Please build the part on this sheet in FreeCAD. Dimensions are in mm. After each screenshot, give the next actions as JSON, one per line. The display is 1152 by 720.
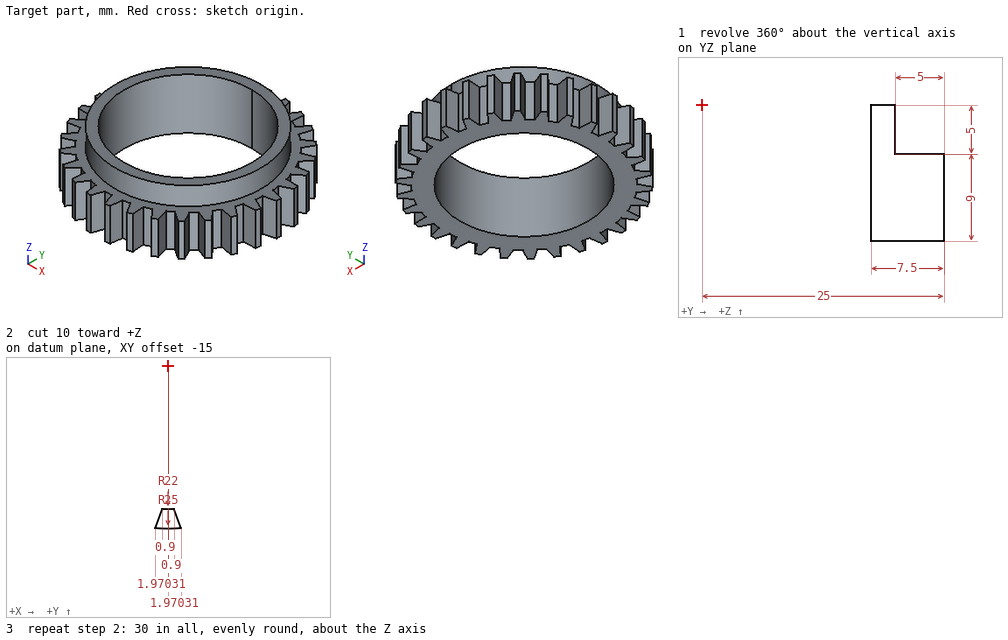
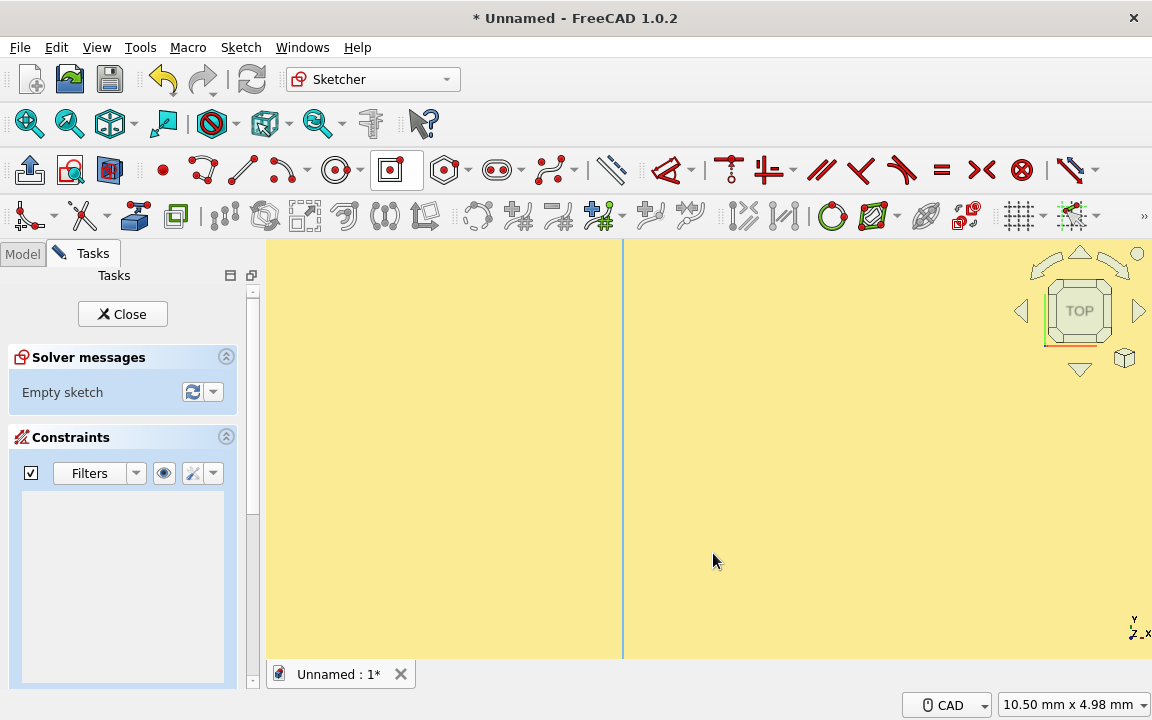
{"action": "left_click", "coordinate": [244, 170]}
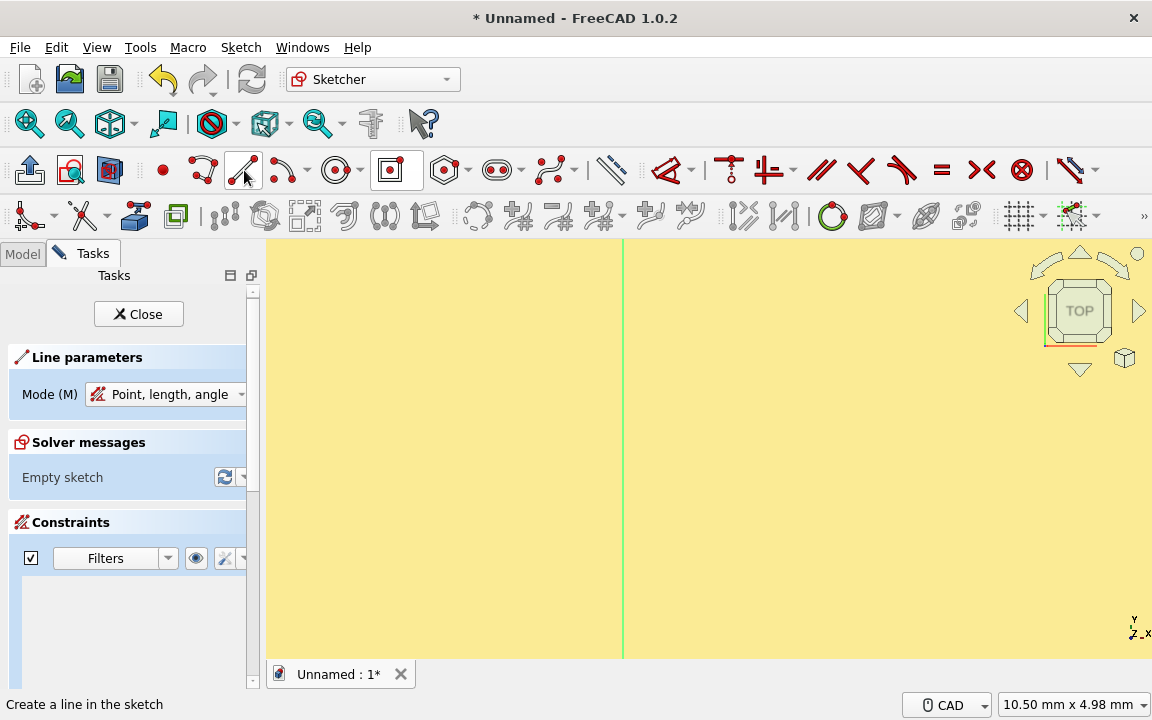
{"action": "left_click", "coordinate": [547, 304]}
{"action": "left_click", "coordinate": [457, 552]}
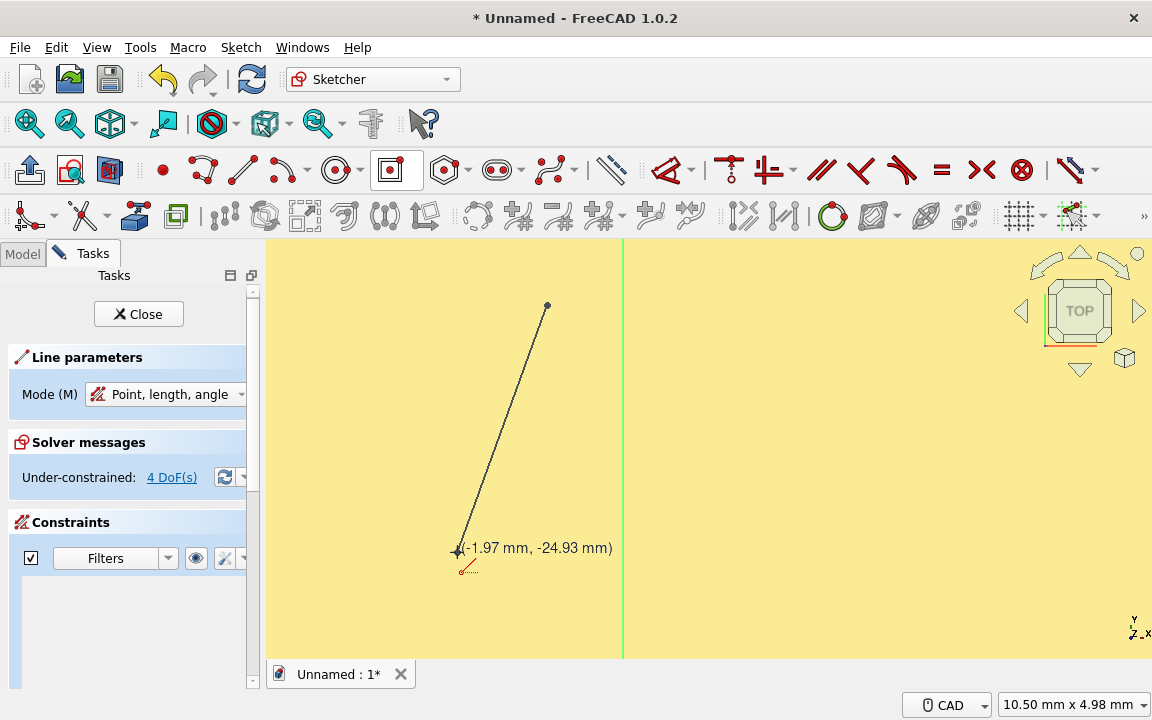
{"action": "left_click", "coordinate": [789, 552]}
{"action": "left_click", "coordinate": [699, 304]}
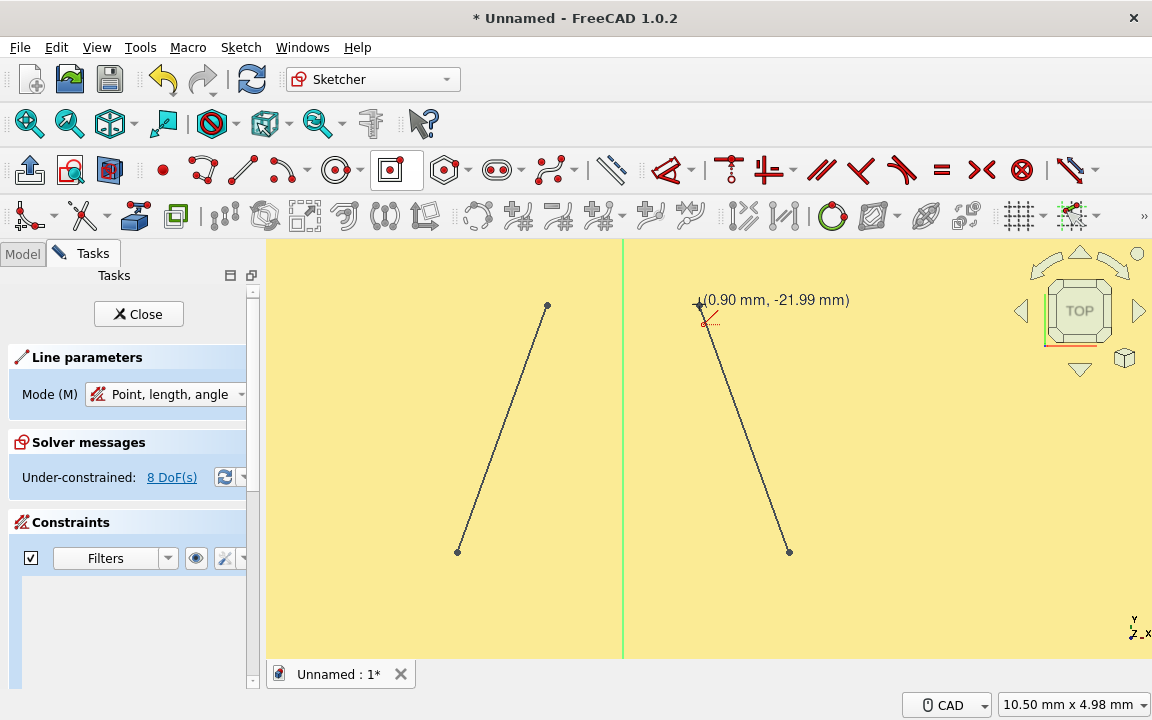
{"action": "left_click", "coordinate": [310, 170]}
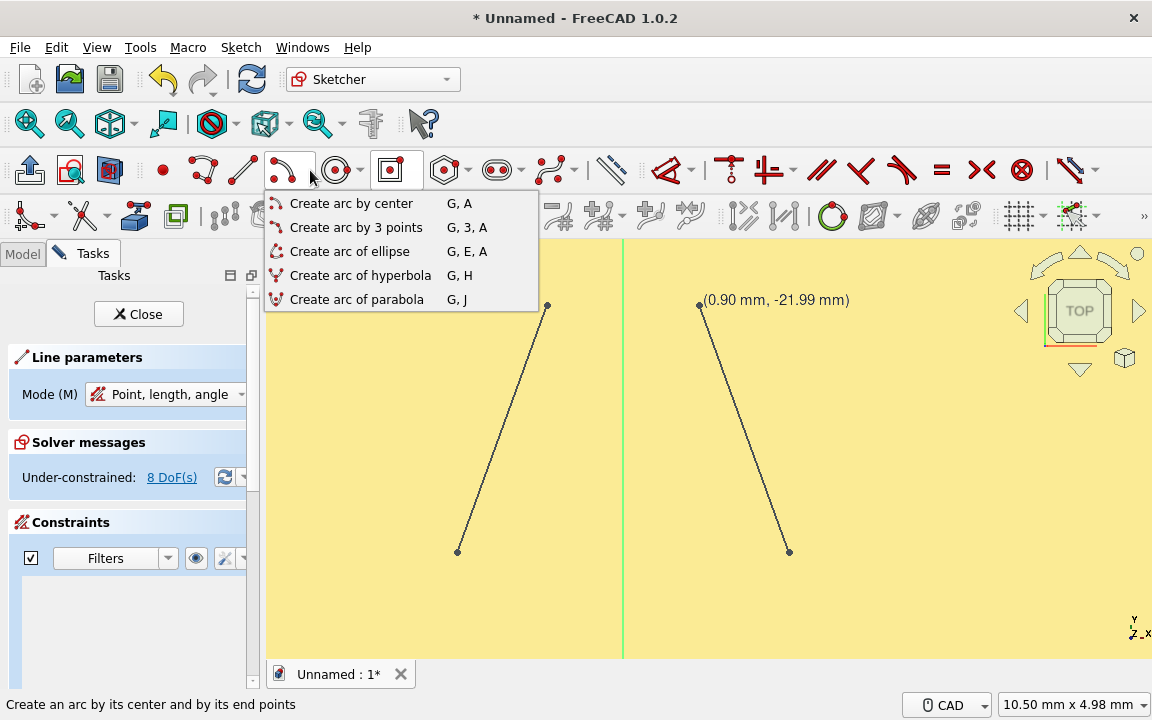
{"action": "left_click", "coordinate": [402, 227]}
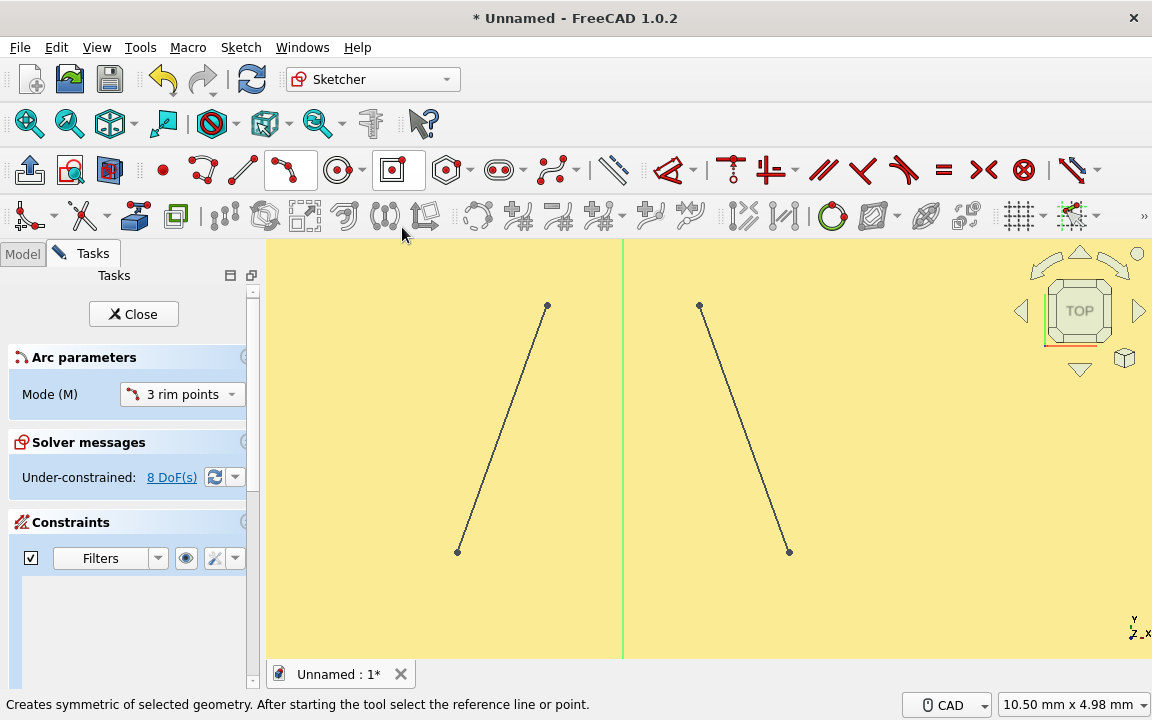
{"action": "left_click", "coordinate": [457, 553]}
{"action": "left_click", "coordinate": [789, 553]}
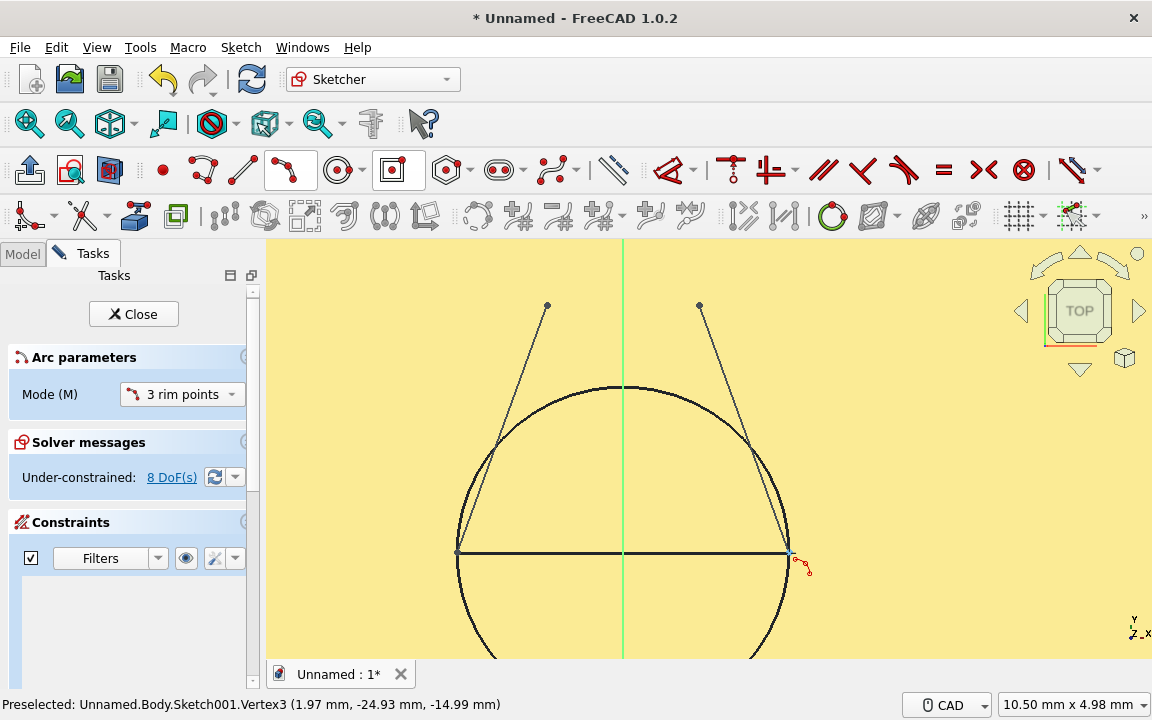
{"action": "scroll", "coordinate": [590, 559], "scroll_direction": "up", "scroll_amount": 5}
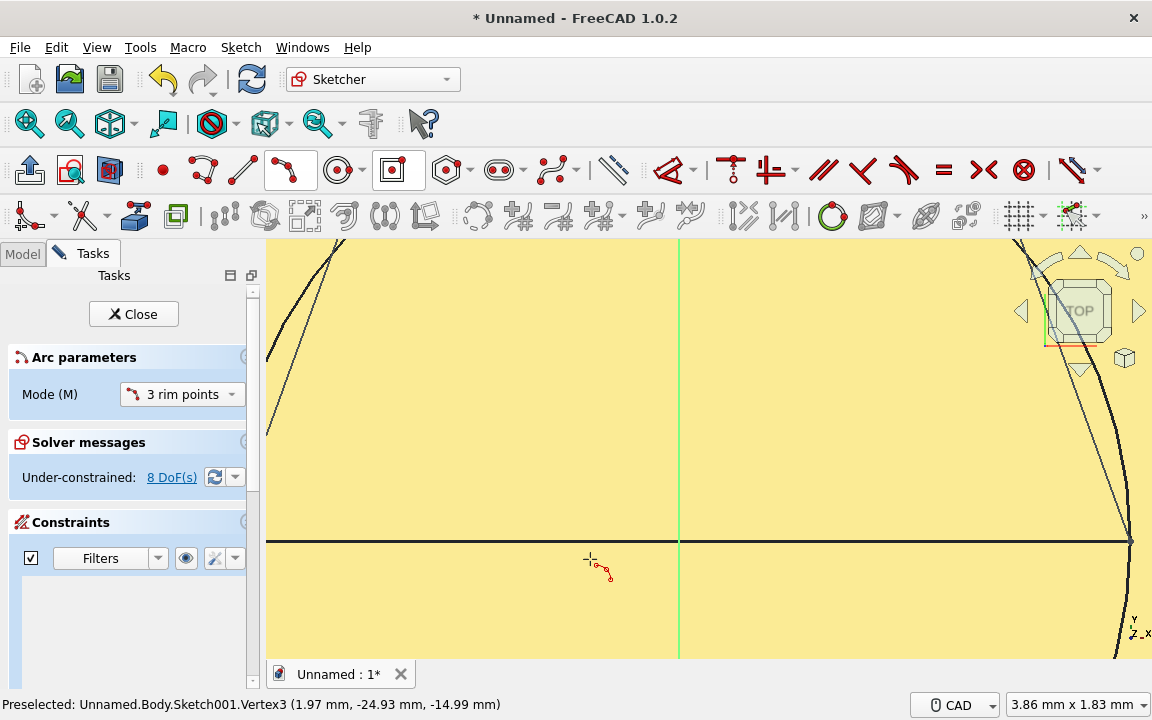
{"action": "left_click", "coordinate": [589, 556]}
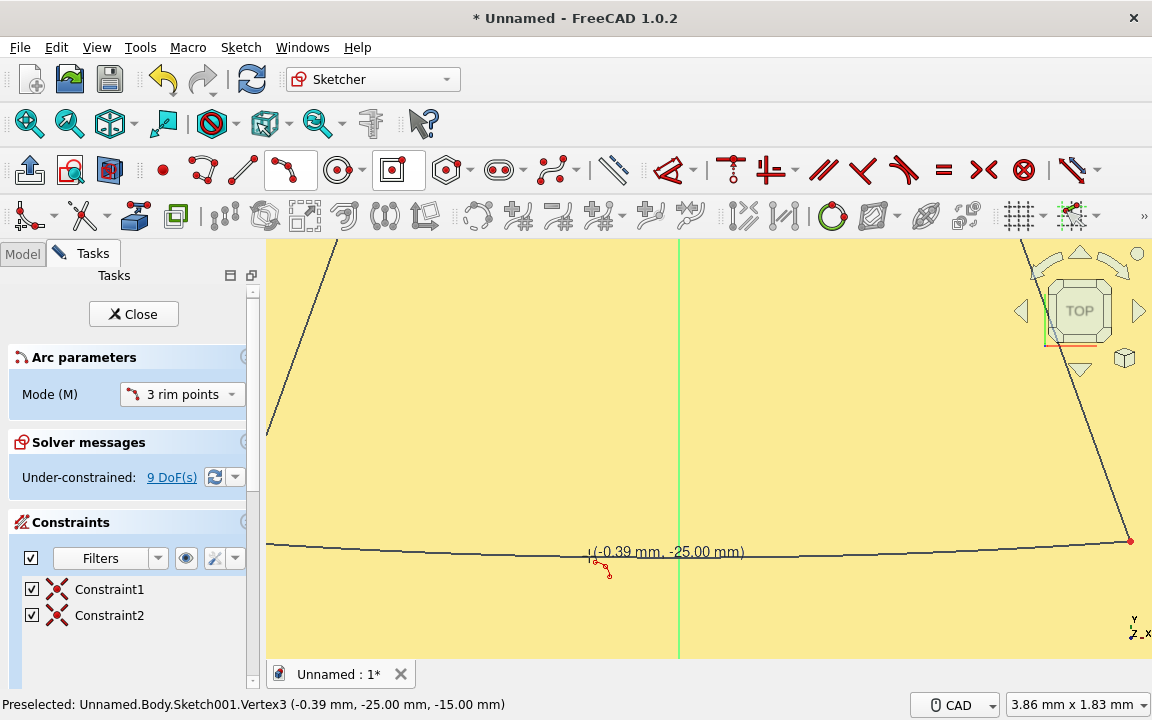
{"action": "scroll", "coordinate": [618, 588], "scroll_direction": "down", "scroll_amount": 5}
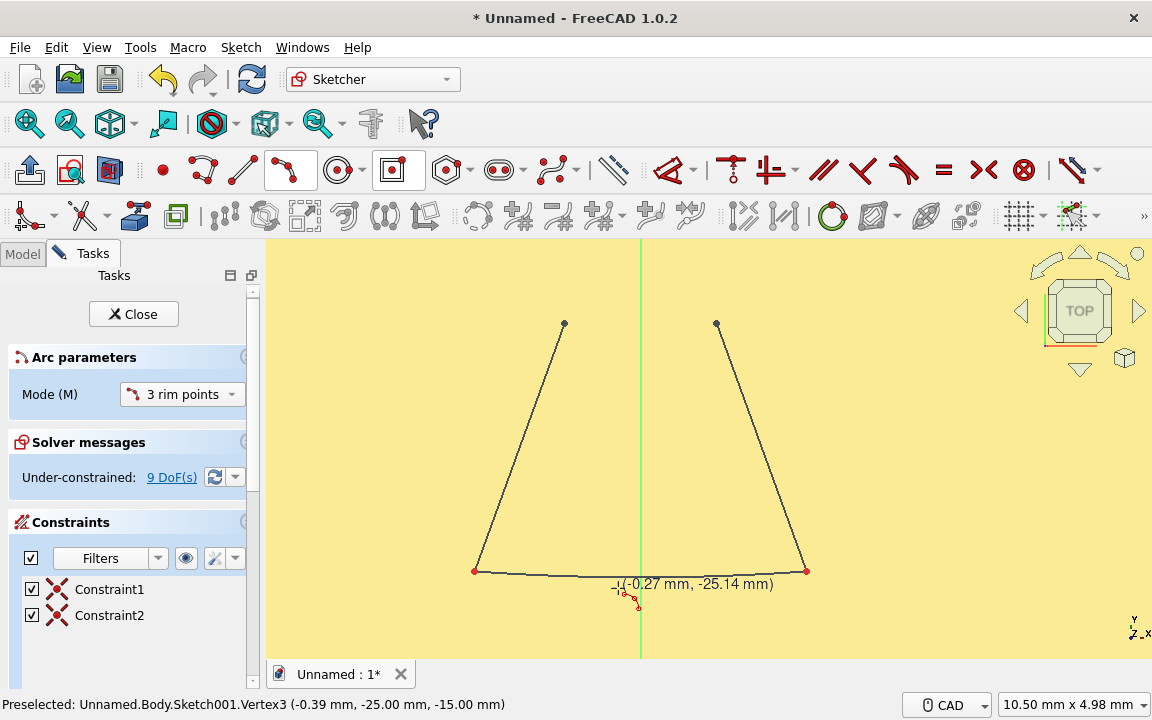
{"action": "left_click", "coordinate": [717, 323]}
{"action": "left_click", "coordinate": [565, 323]}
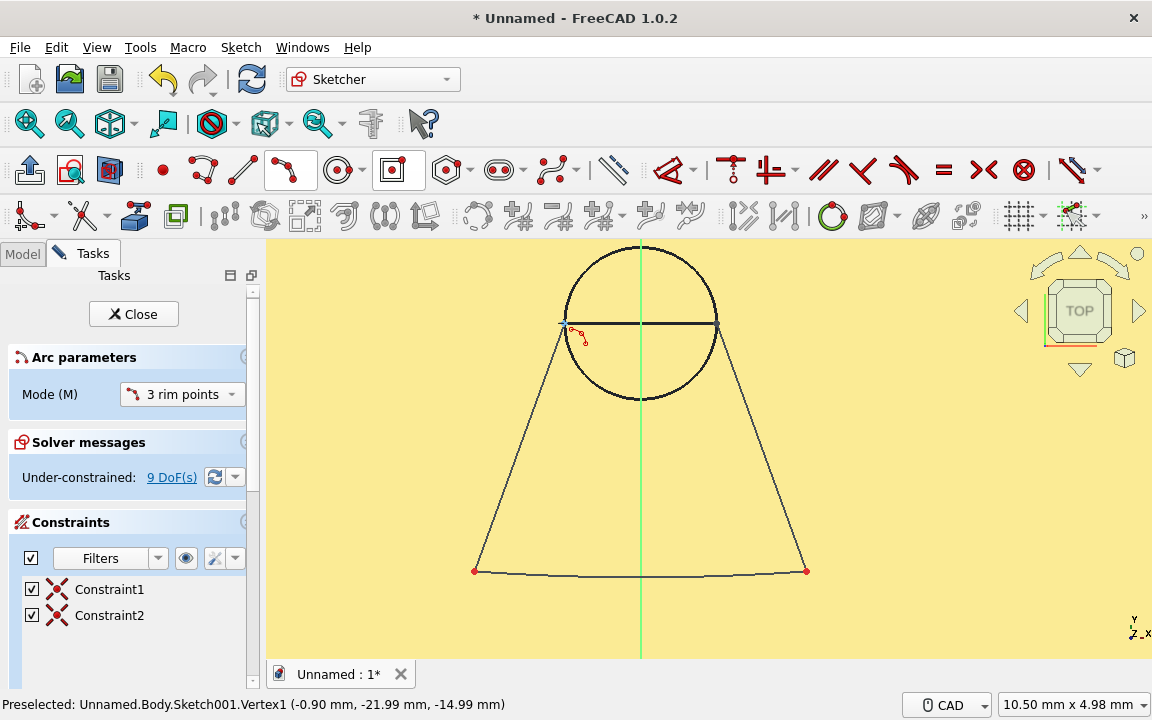
{"action": "scroll", "coordinate": [626, 324], "scroll_direction": "up", "scroll_amount": 12}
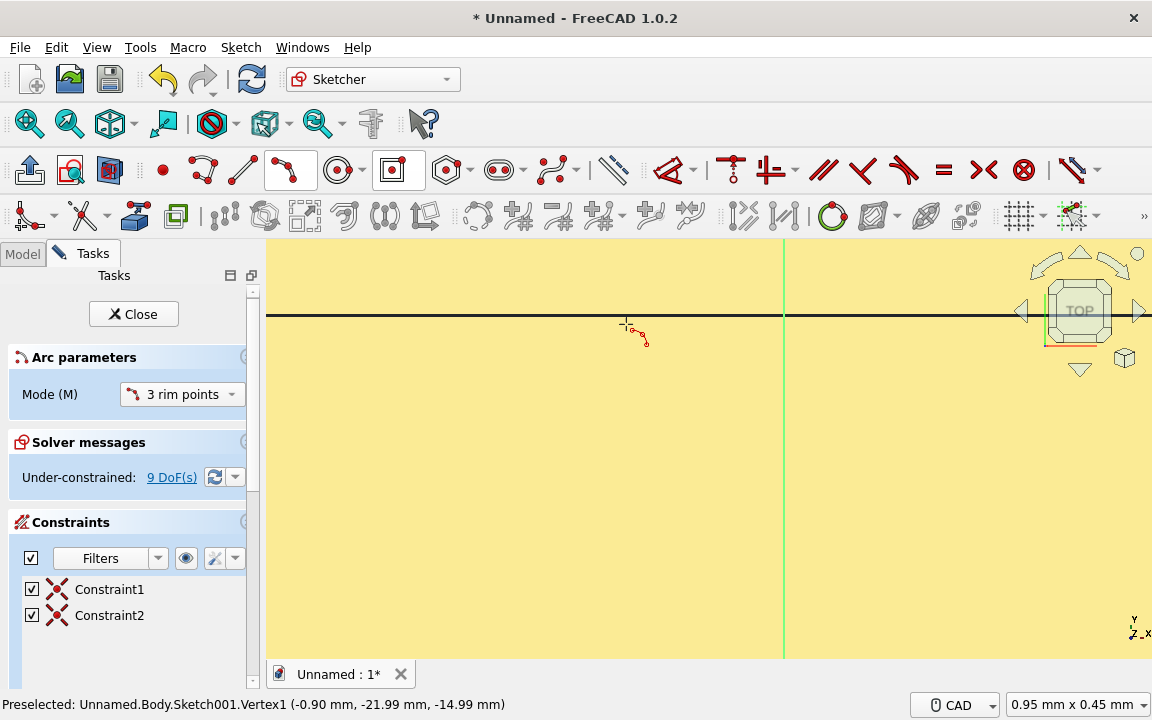
{"action": "left_click", "coordinate": [617, 322]}
{"action": "key", "text": "Escape"}